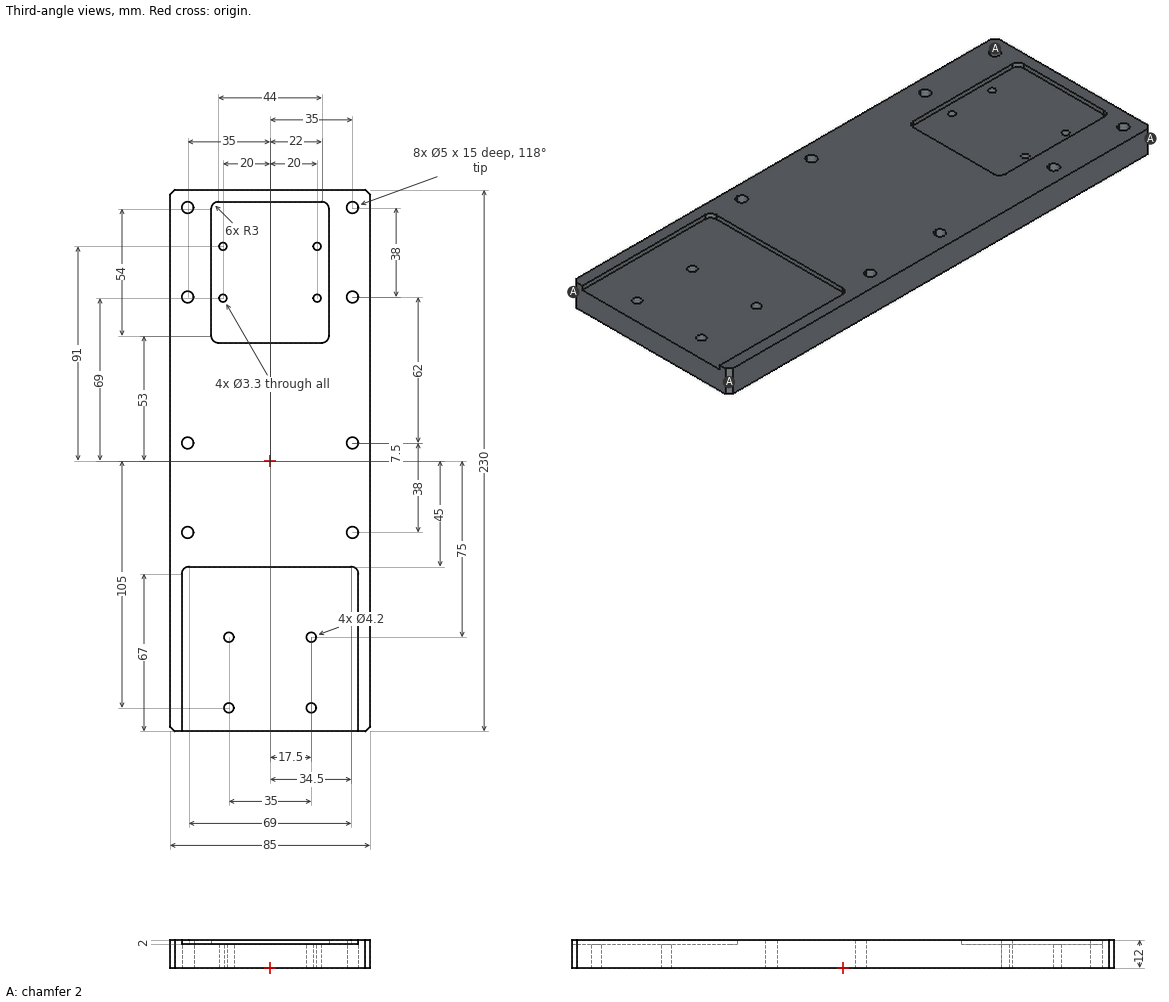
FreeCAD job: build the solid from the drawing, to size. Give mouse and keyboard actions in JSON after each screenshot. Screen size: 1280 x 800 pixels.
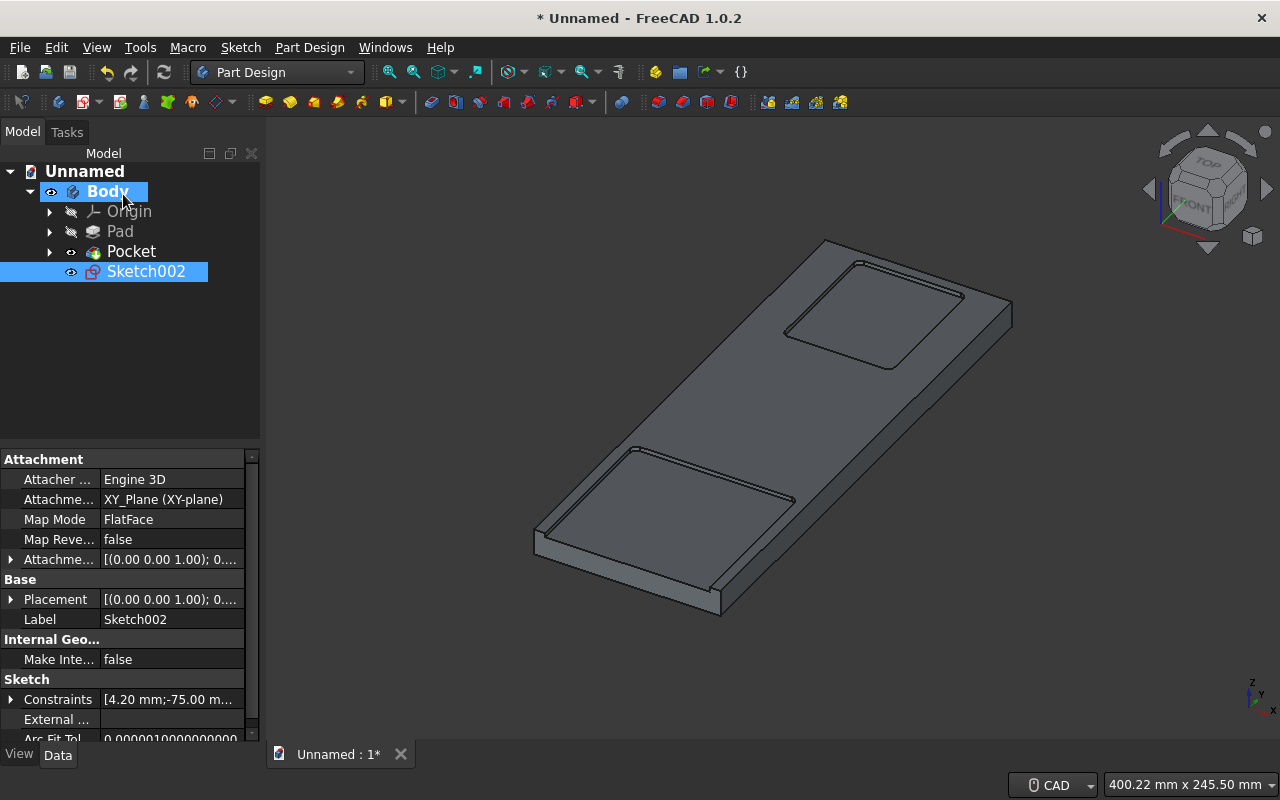
{"action": "left_click", "coordinate": [432, 102]}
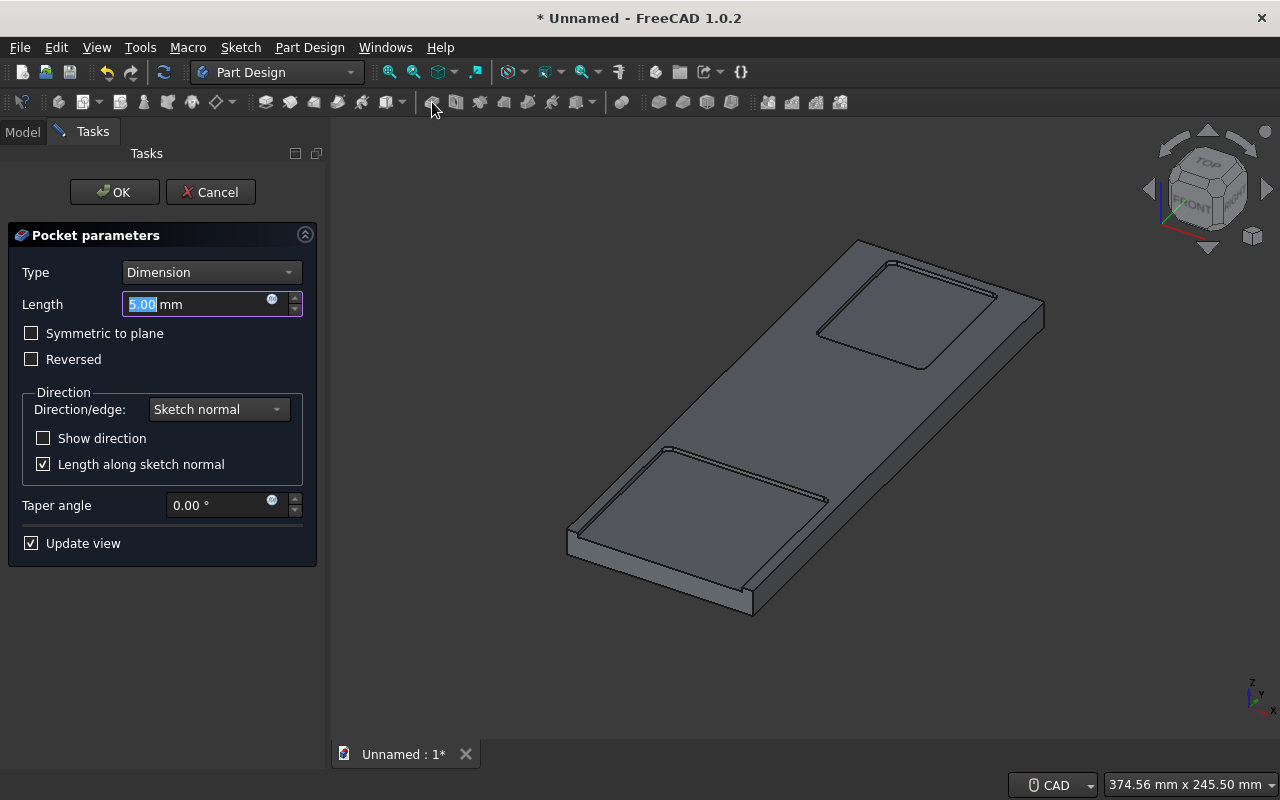
{"action": "left_click", "coordinate": [212, 272]}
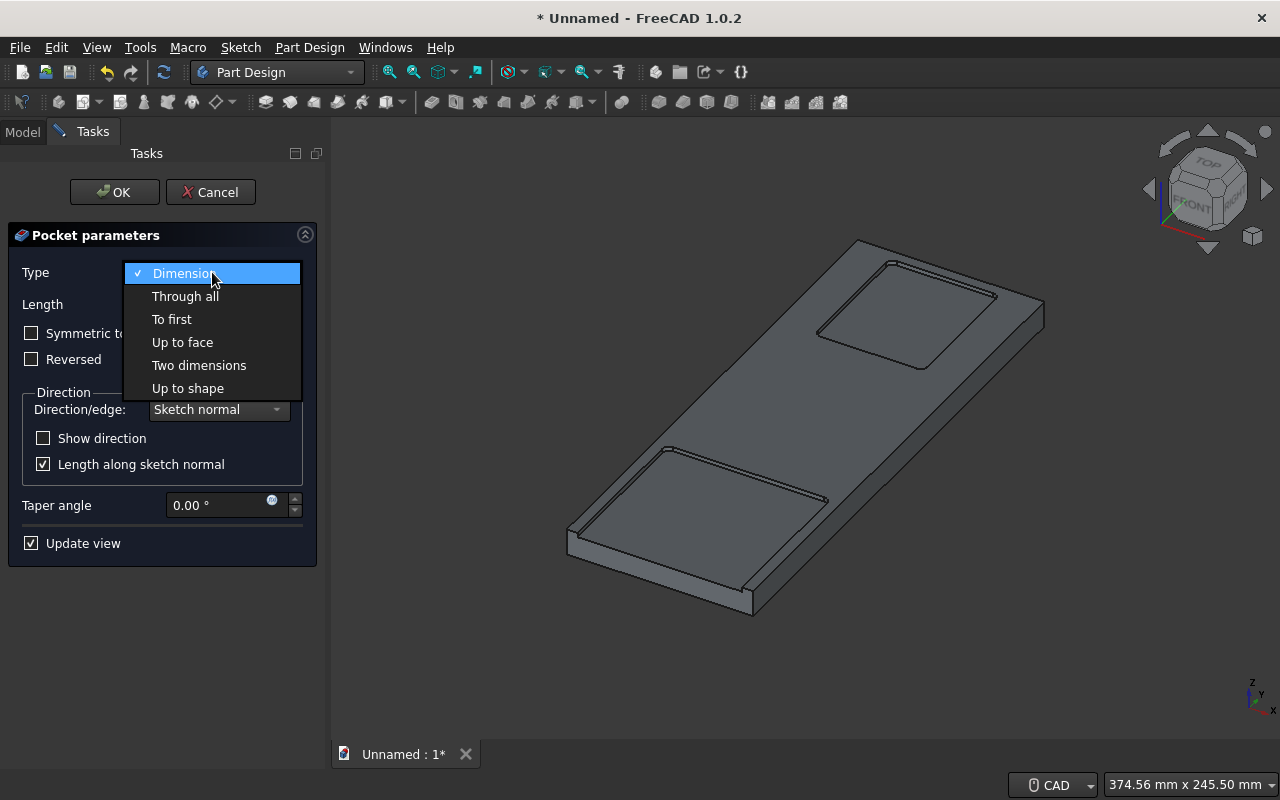
{"action": "left_click", "coordinate": [212, 296]}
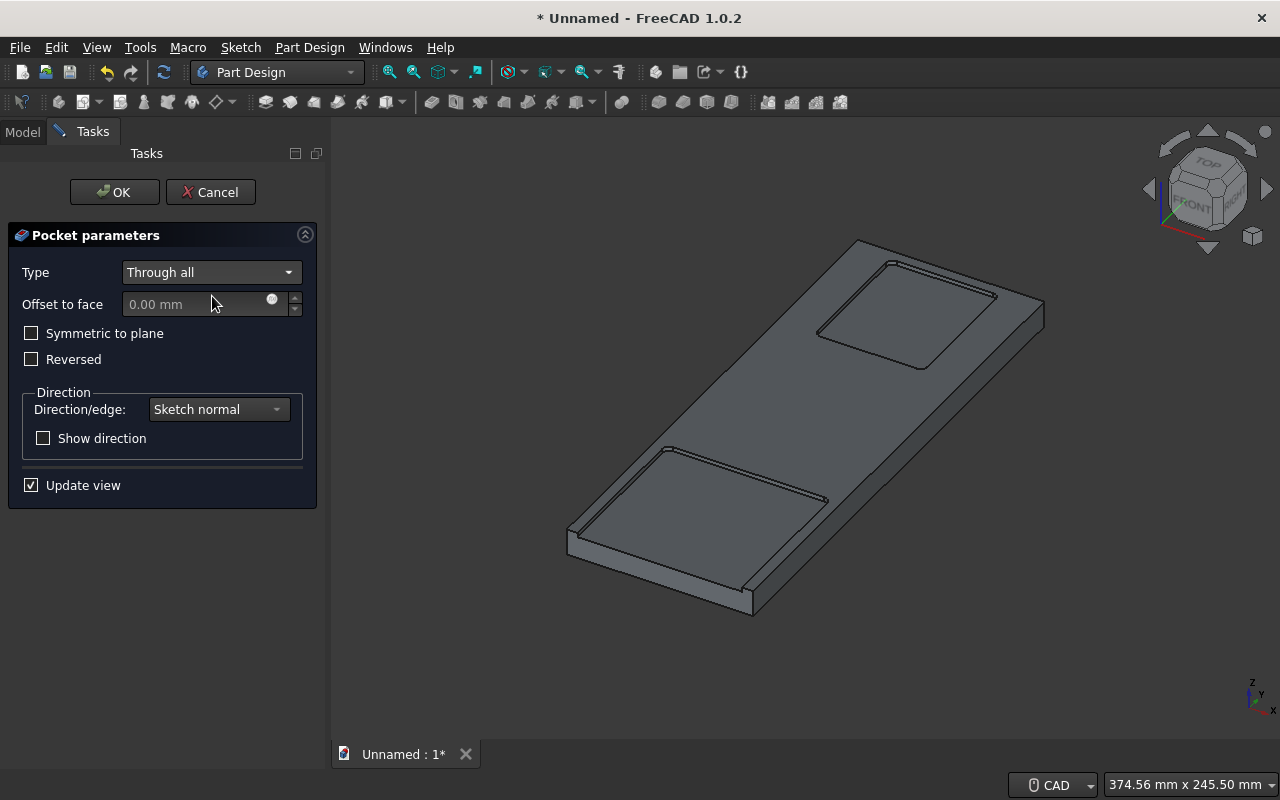
{"action": "left_click", "coordinate": [30, 359]}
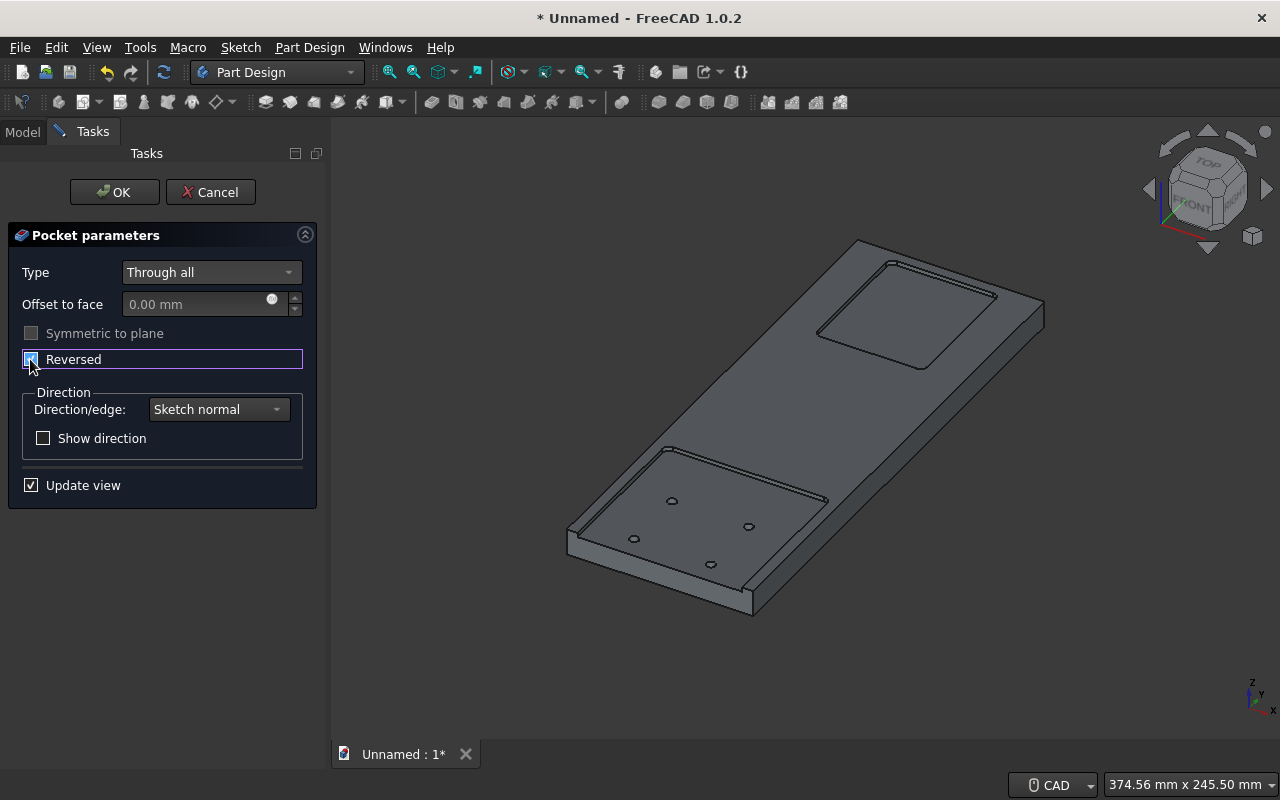
{"action": "left_click", "coordinate": [115, 192]}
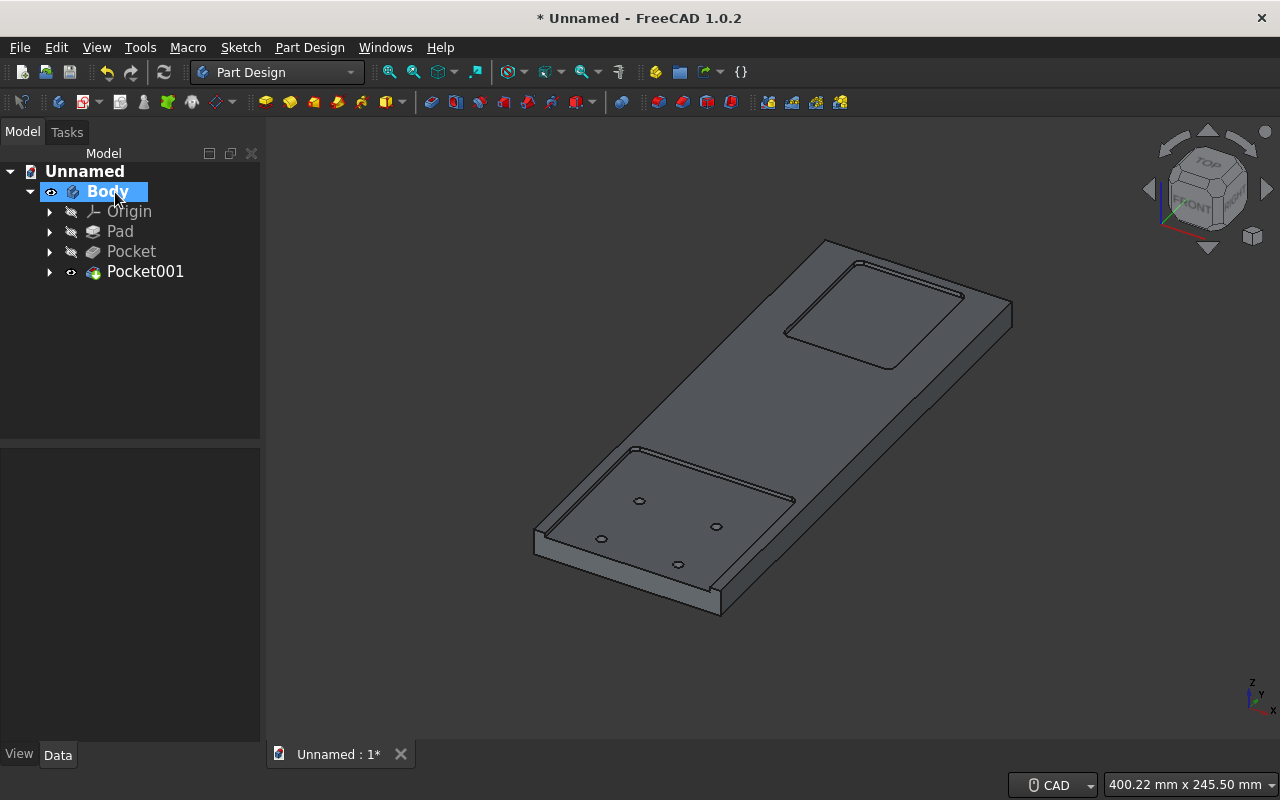
{"action": "left_click", "coordinate": [773, 415]}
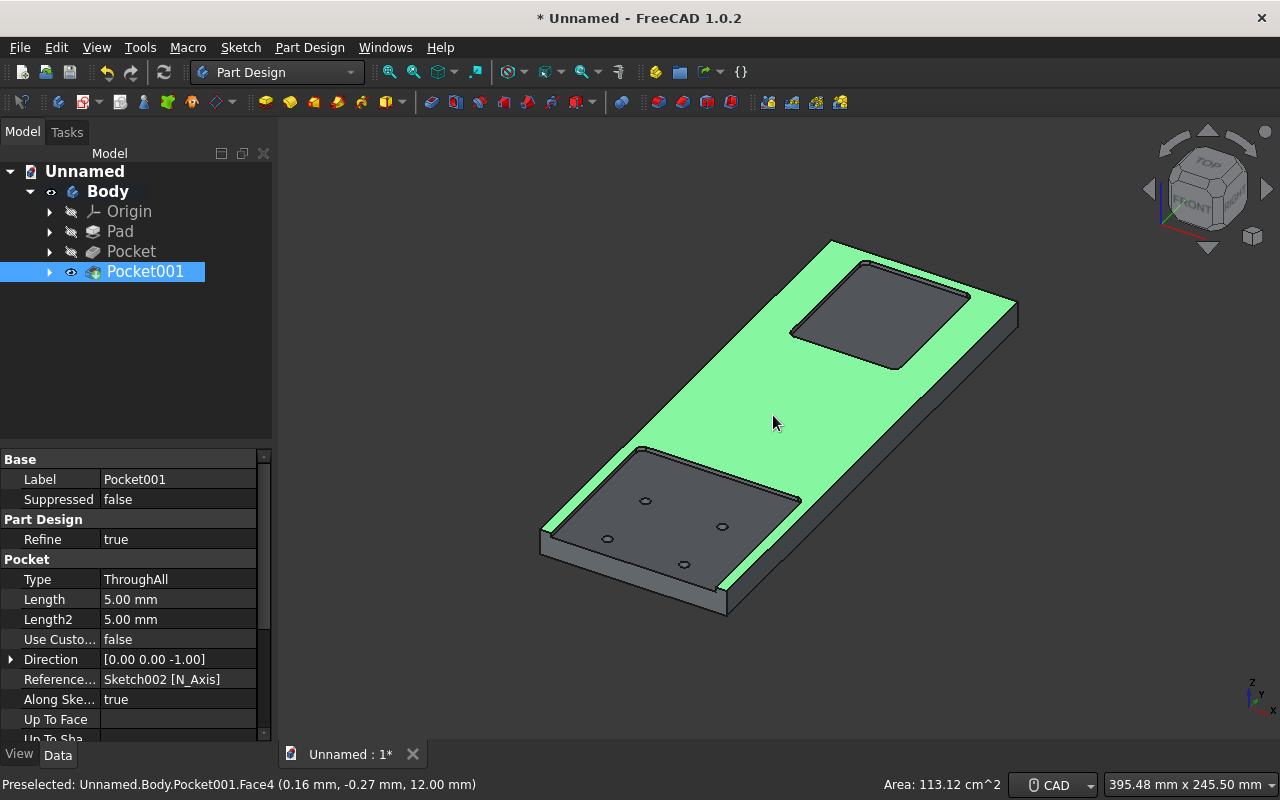
{"action": "left_click", "coordinate": [84, 102]}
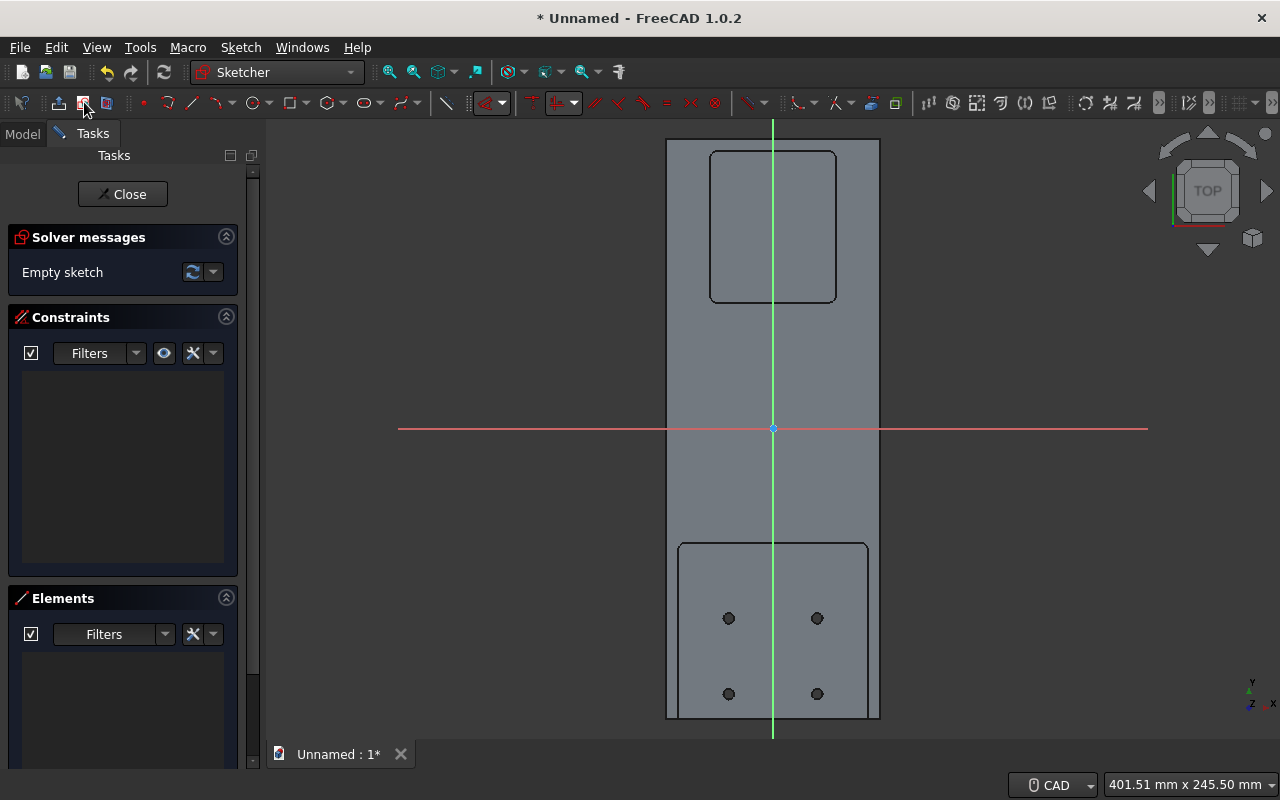
{"action": "scroll", "coordinate": [856, 170], "scroll_direction": "up", "scroll_amount": 3}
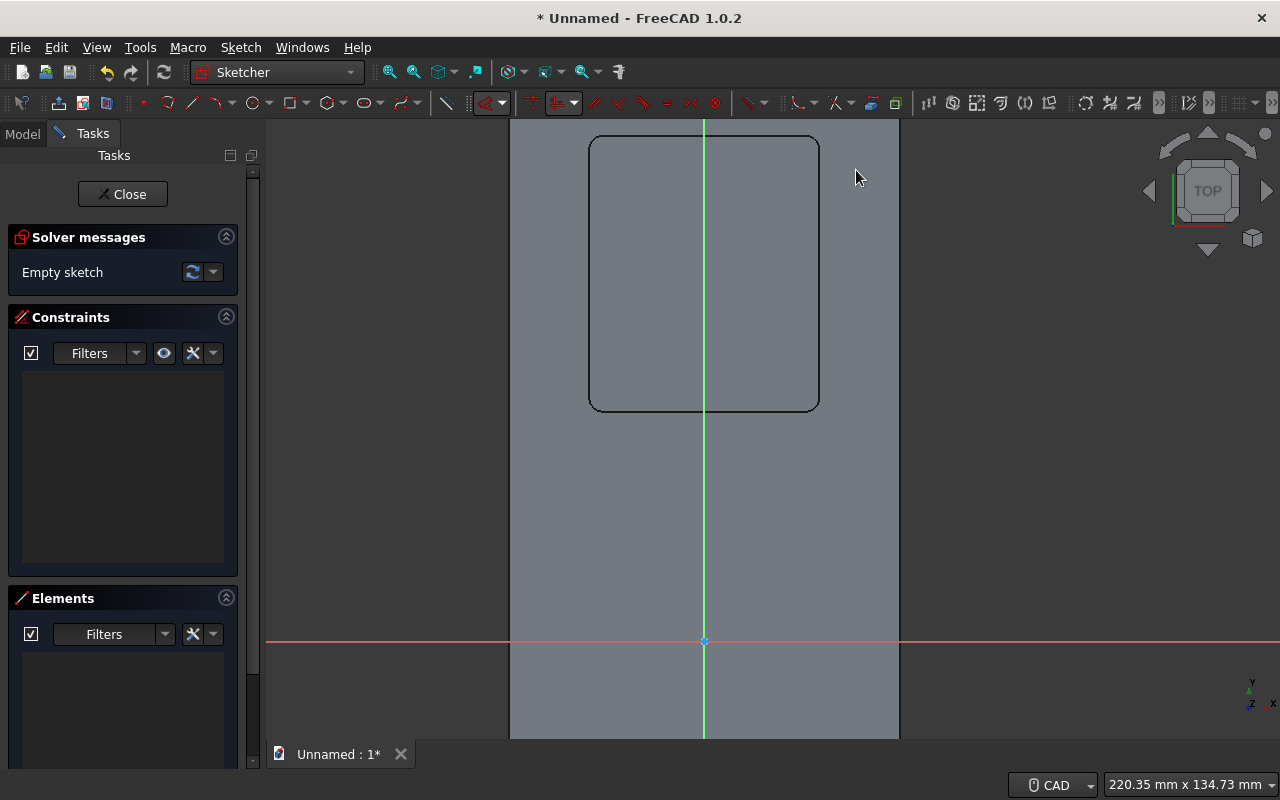
{"action": "key", "text": "g c"}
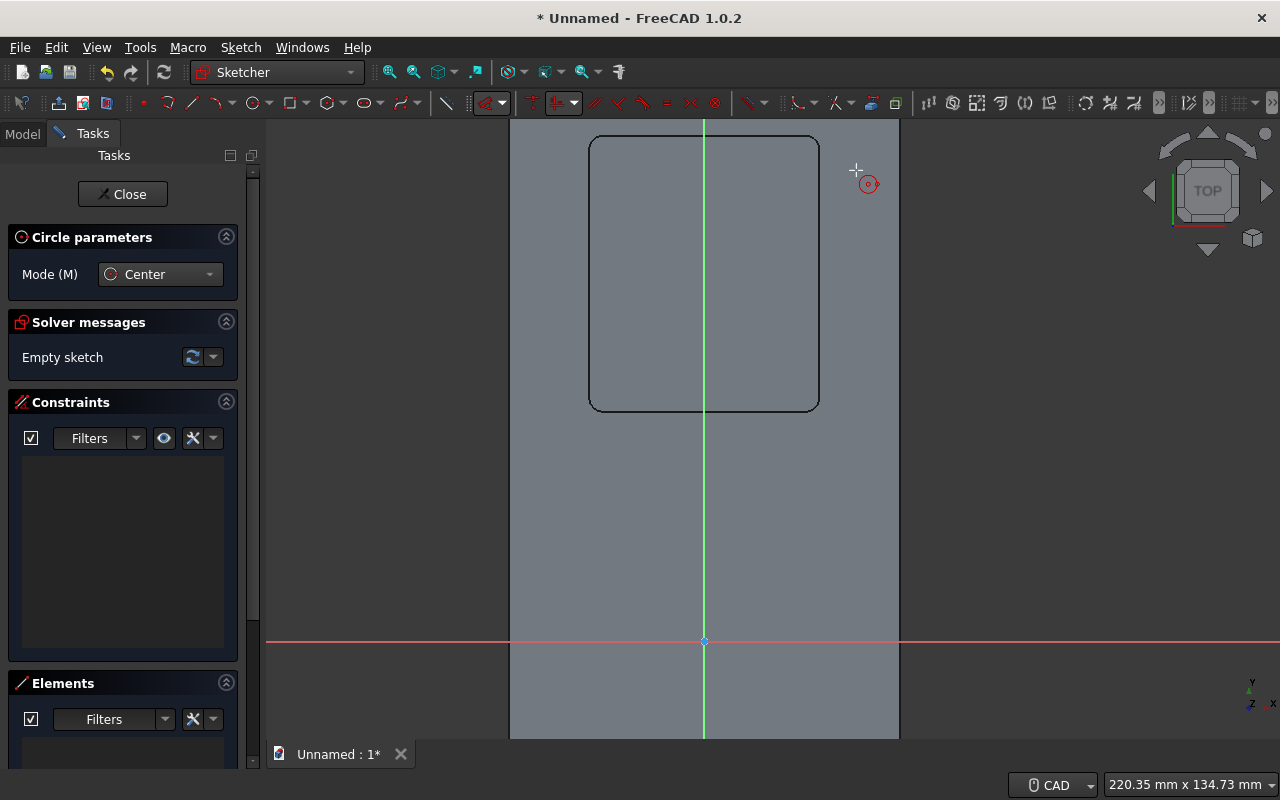
{"action": "scroll", "coordinate": [612, 324], "scroll_direction": "up", "scroll_amount": 6}